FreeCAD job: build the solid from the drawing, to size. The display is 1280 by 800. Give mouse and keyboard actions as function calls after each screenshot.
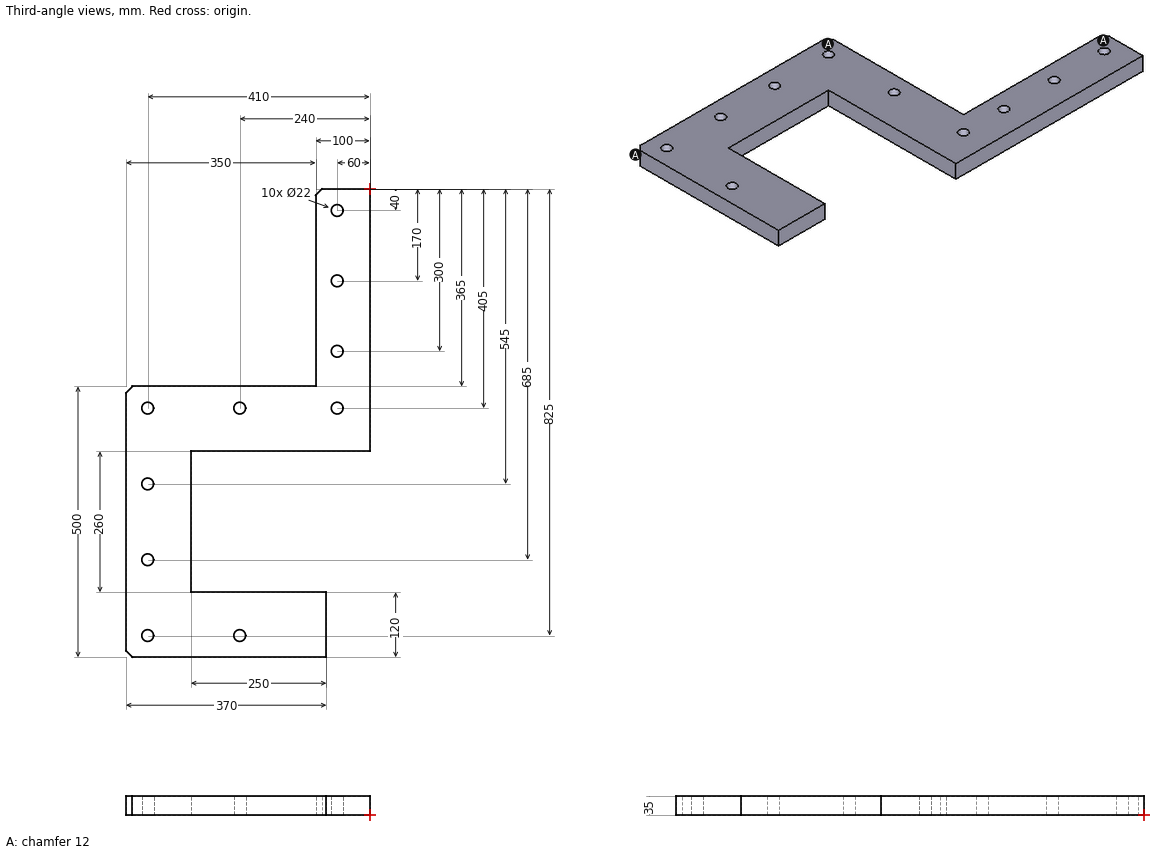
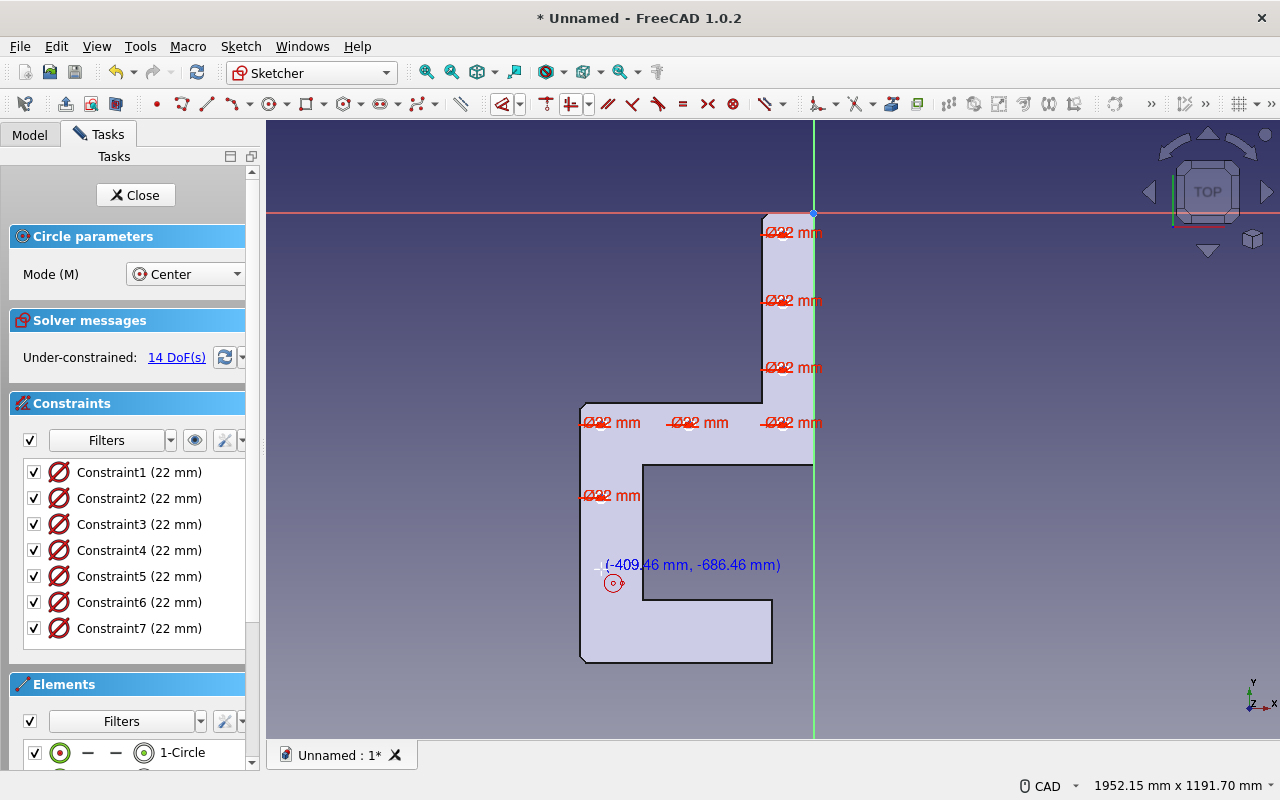
click(601, 569)
move(605, 565)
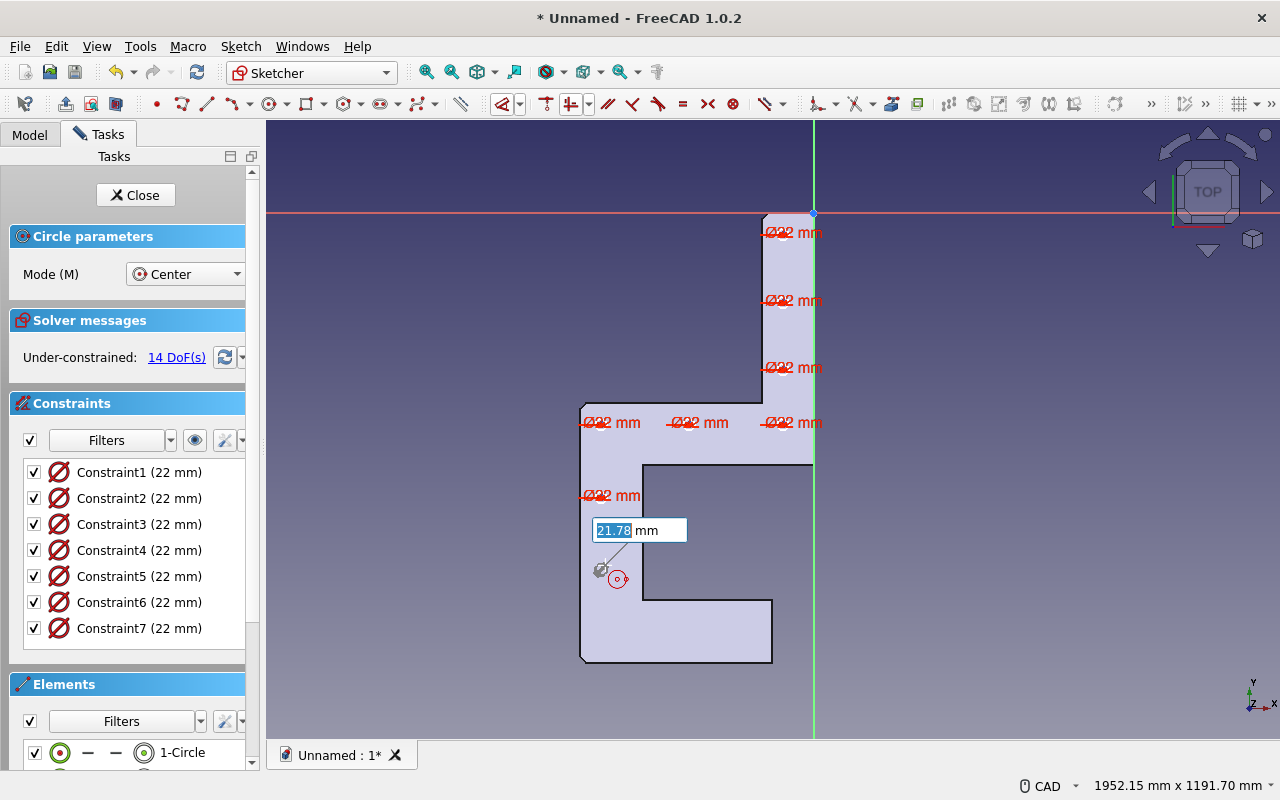
text(22)
key(Return)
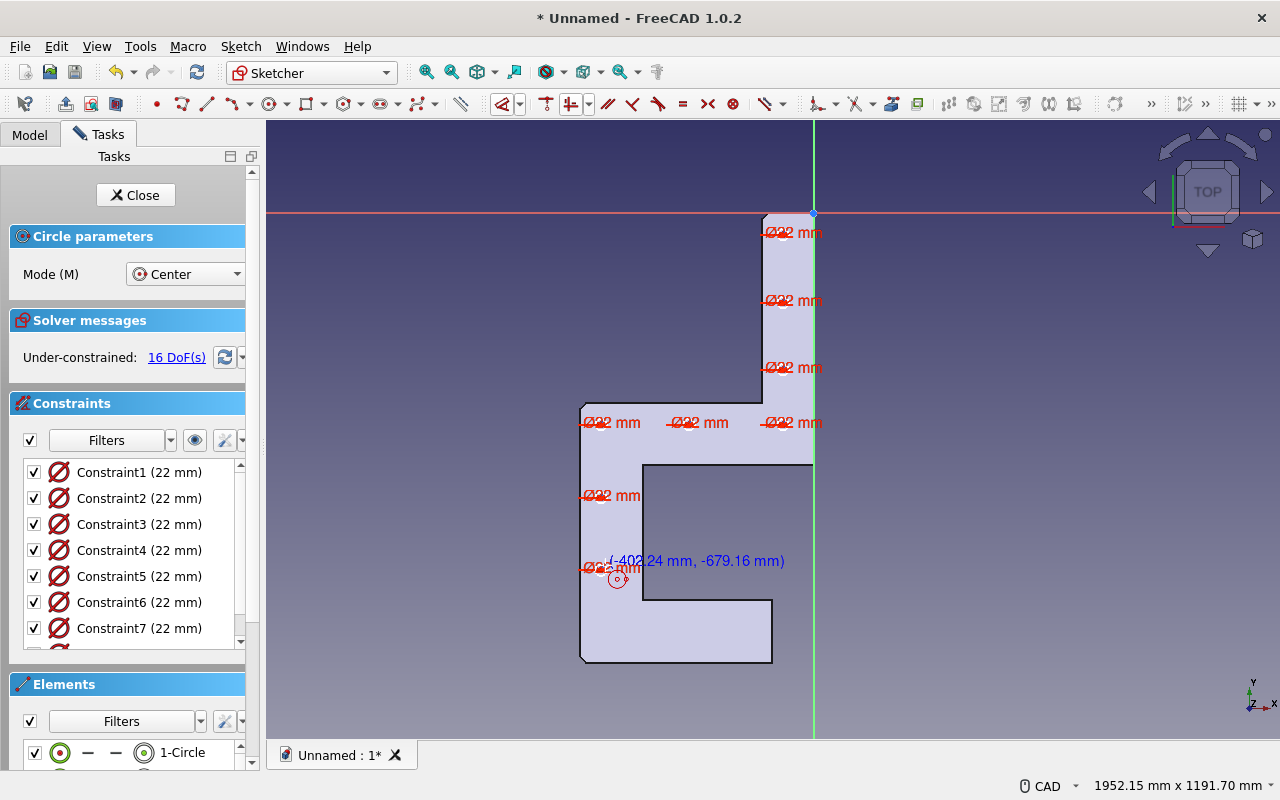
scroll(601, 642, up, 7)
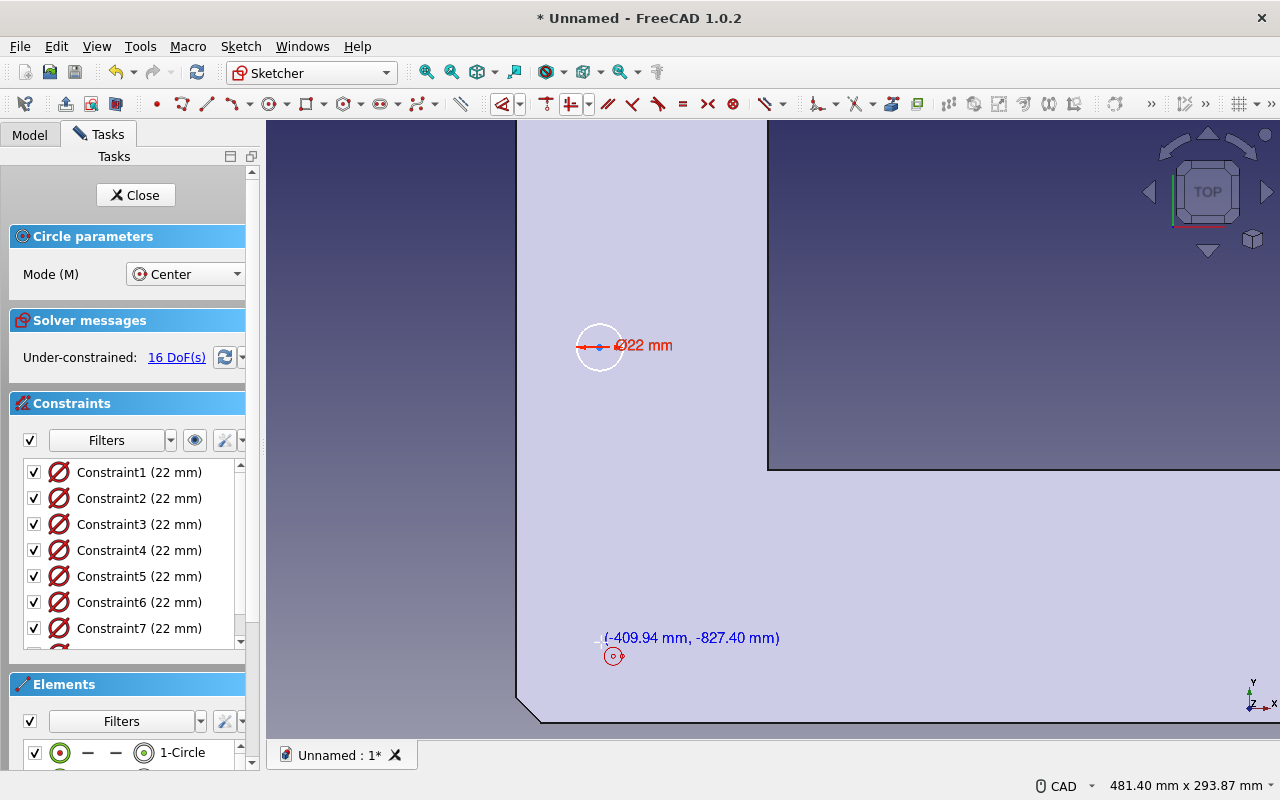
scroll(601, 642, down, 7)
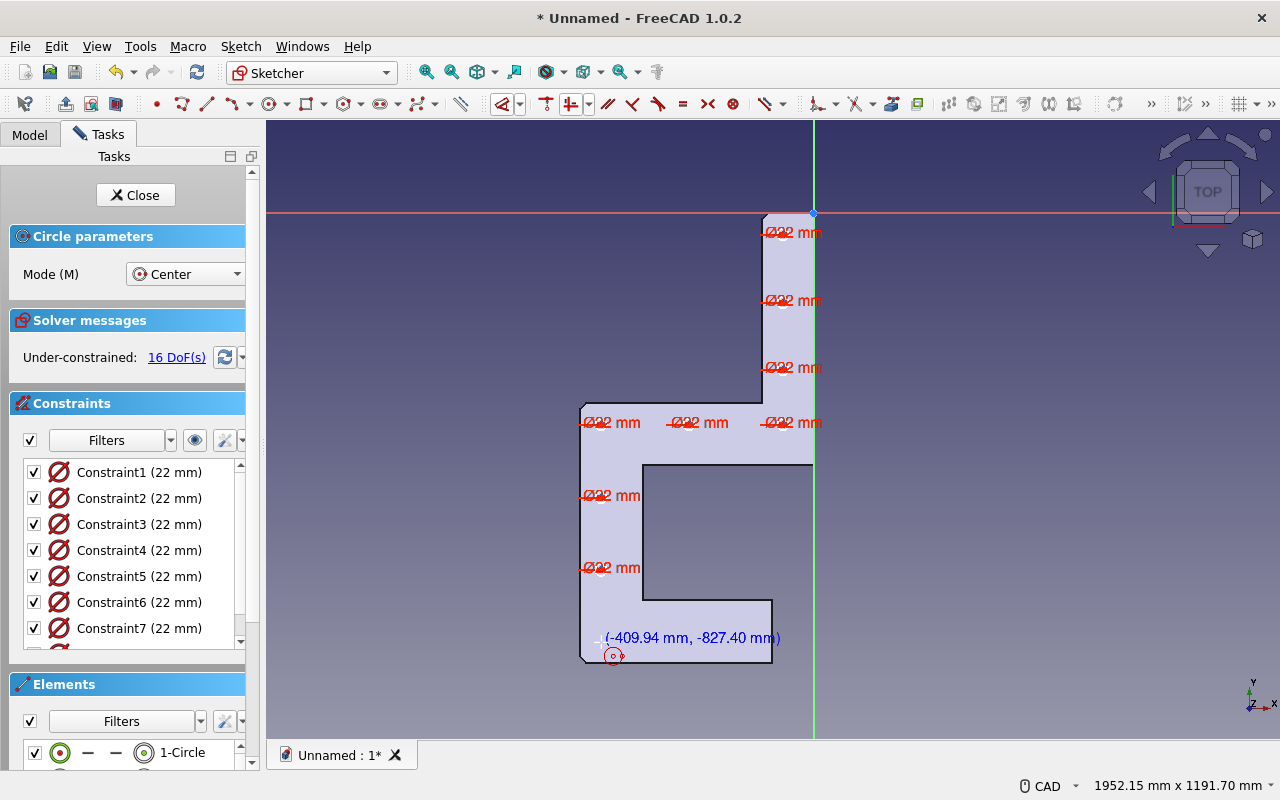
click(601, 642)
move(605, 638)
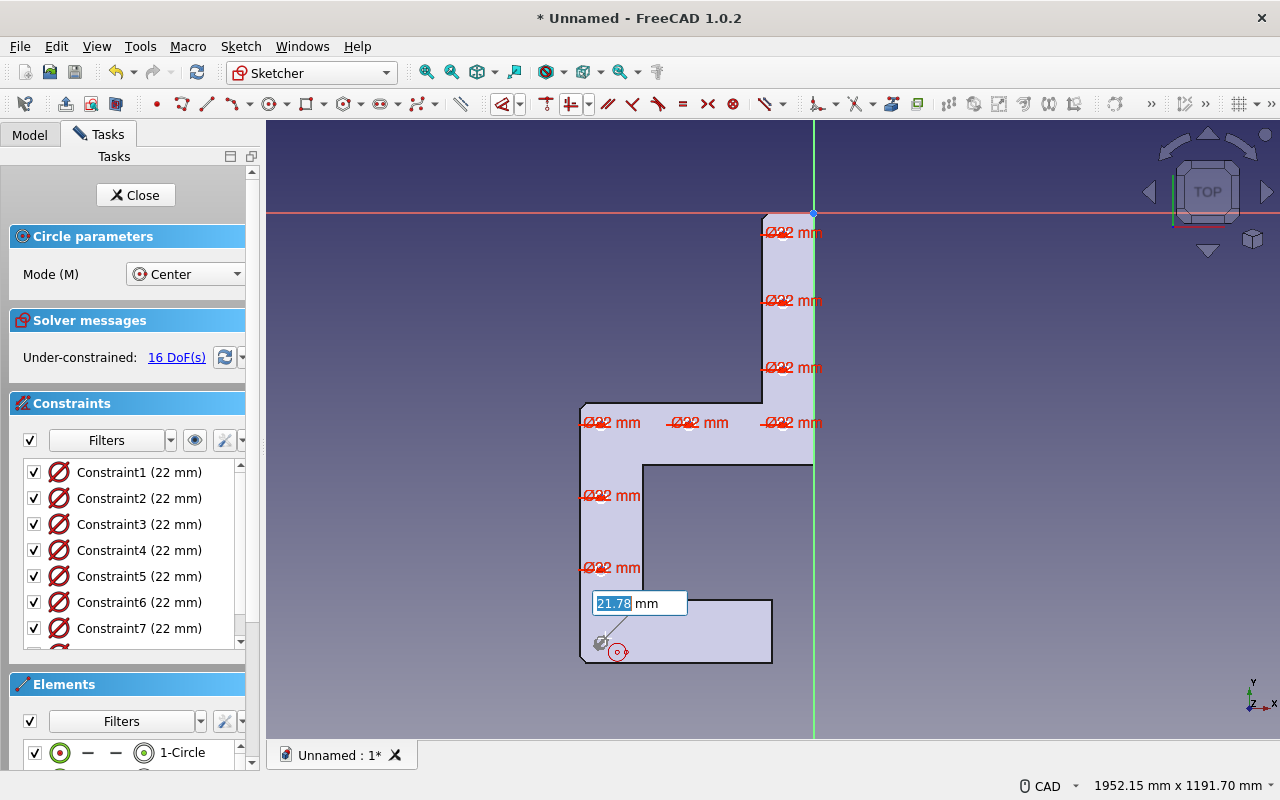
text(22)
key(Return)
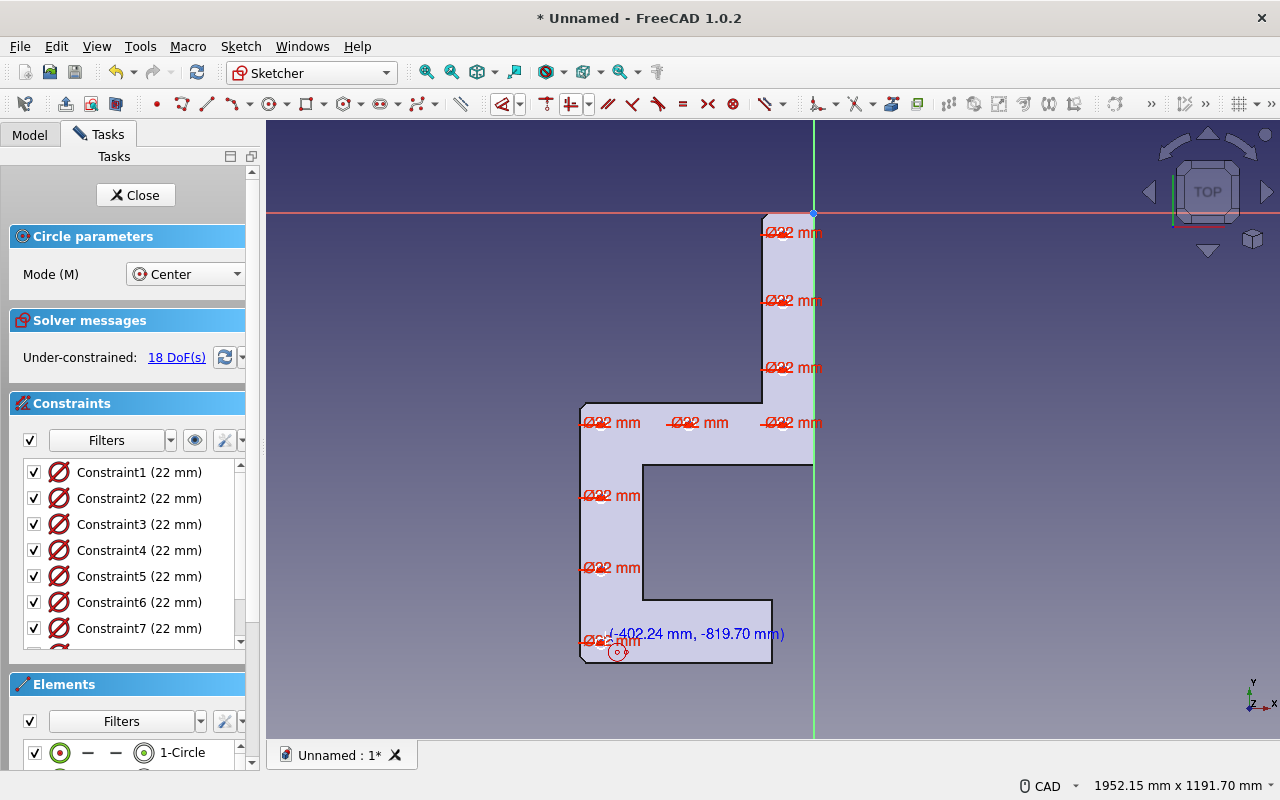
scroll(689, 642, up, 7)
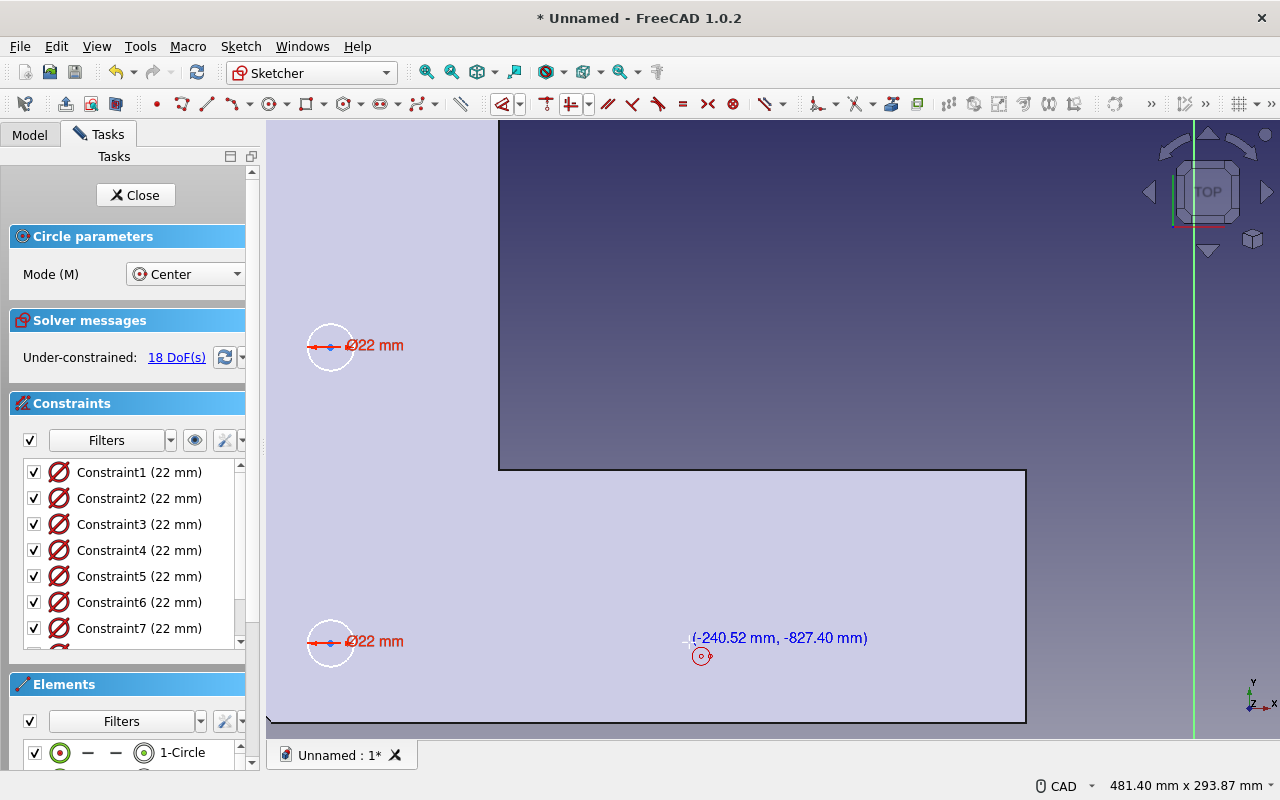
scroll(689, 642, down, 7)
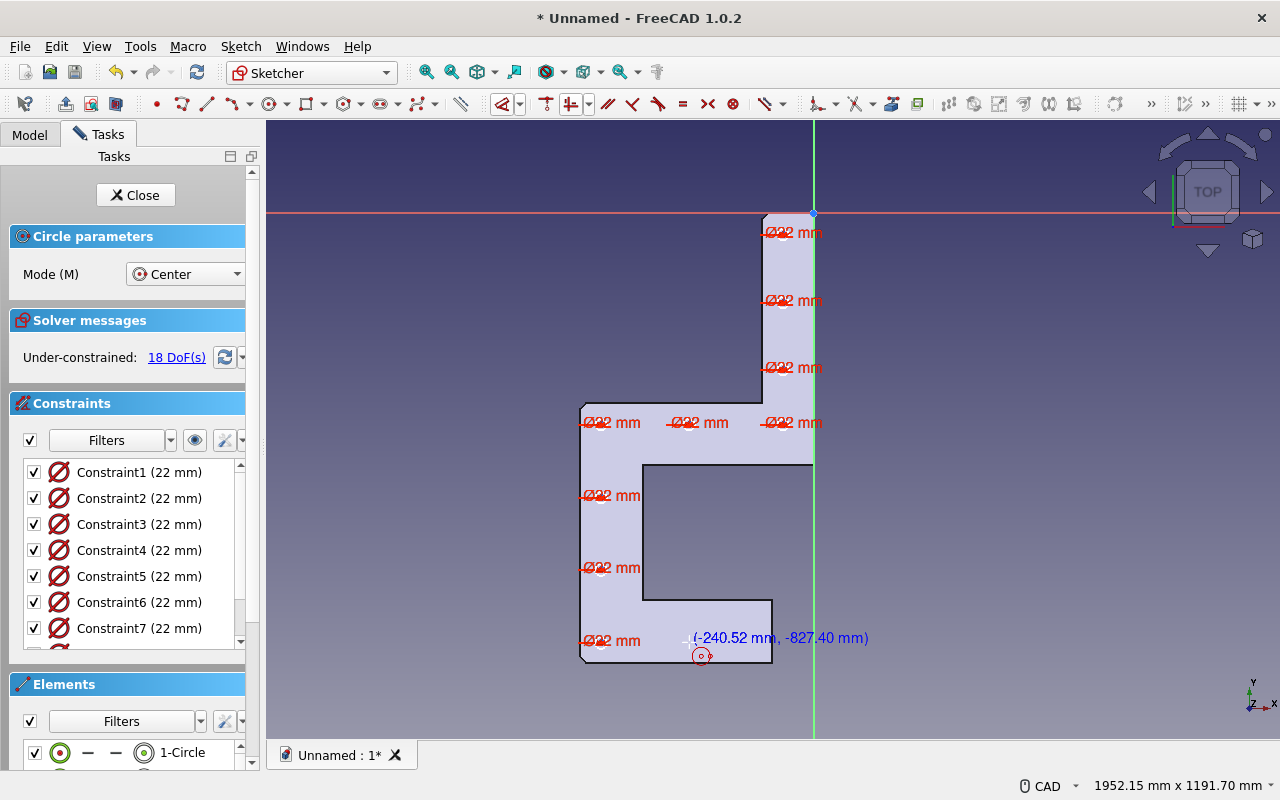
click(689, 642)
move(693, 638)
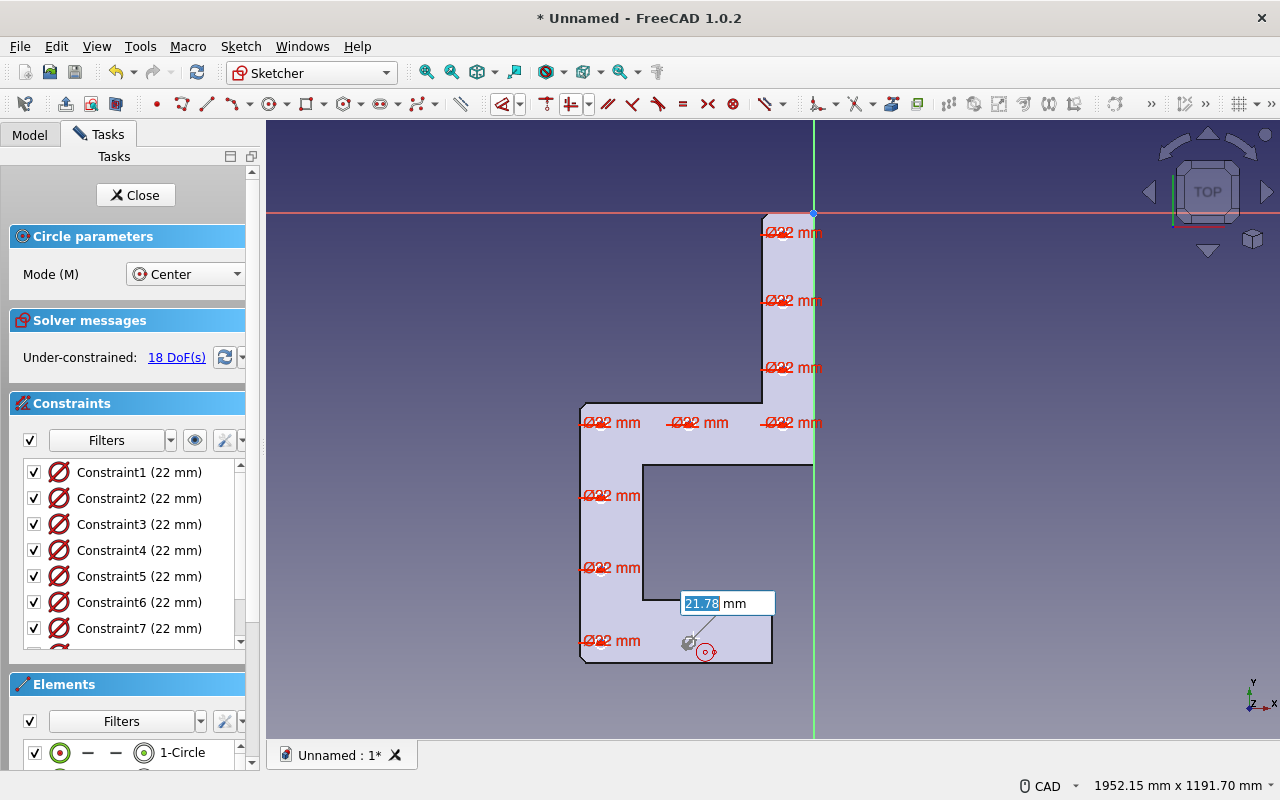
text(22)
key(Return)
key(Escape)